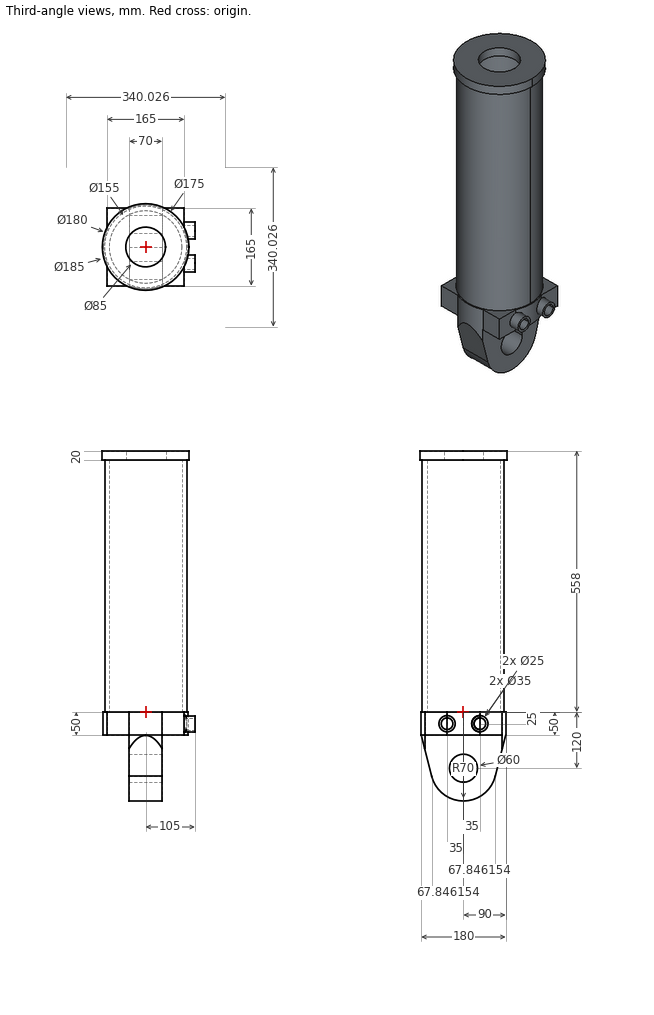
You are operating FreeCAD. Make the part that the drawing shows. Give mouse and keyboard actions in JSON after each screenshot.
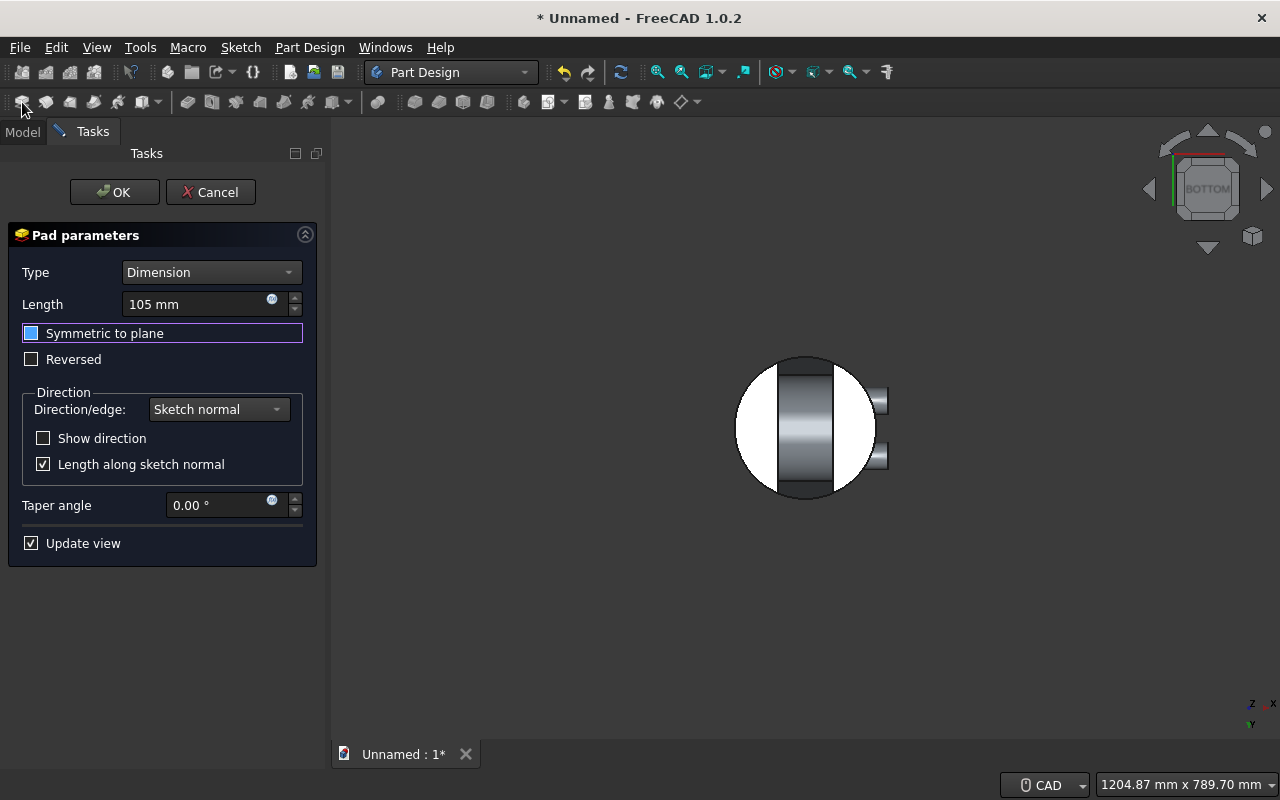
{"action": "left_click", "coordinate": [115, 192]}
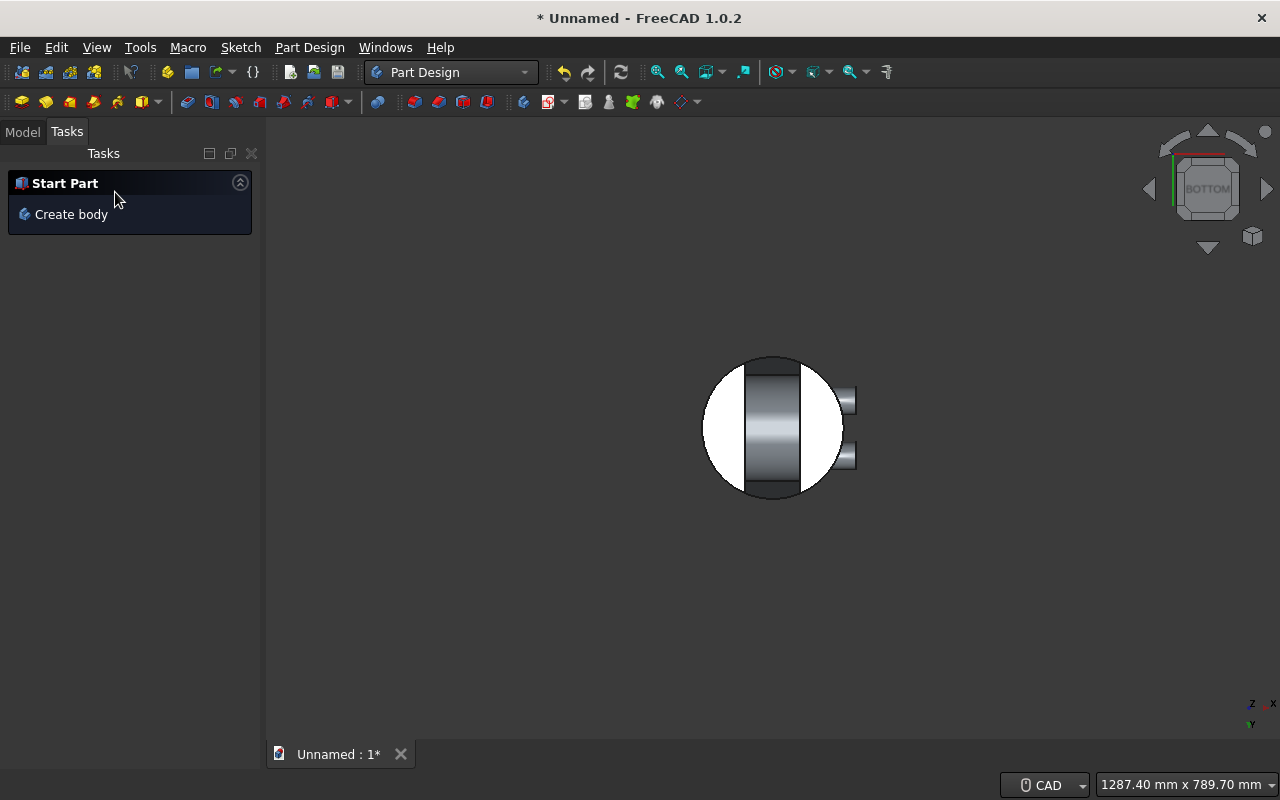
{"action": "left_click", "coordinate": [658, 72]}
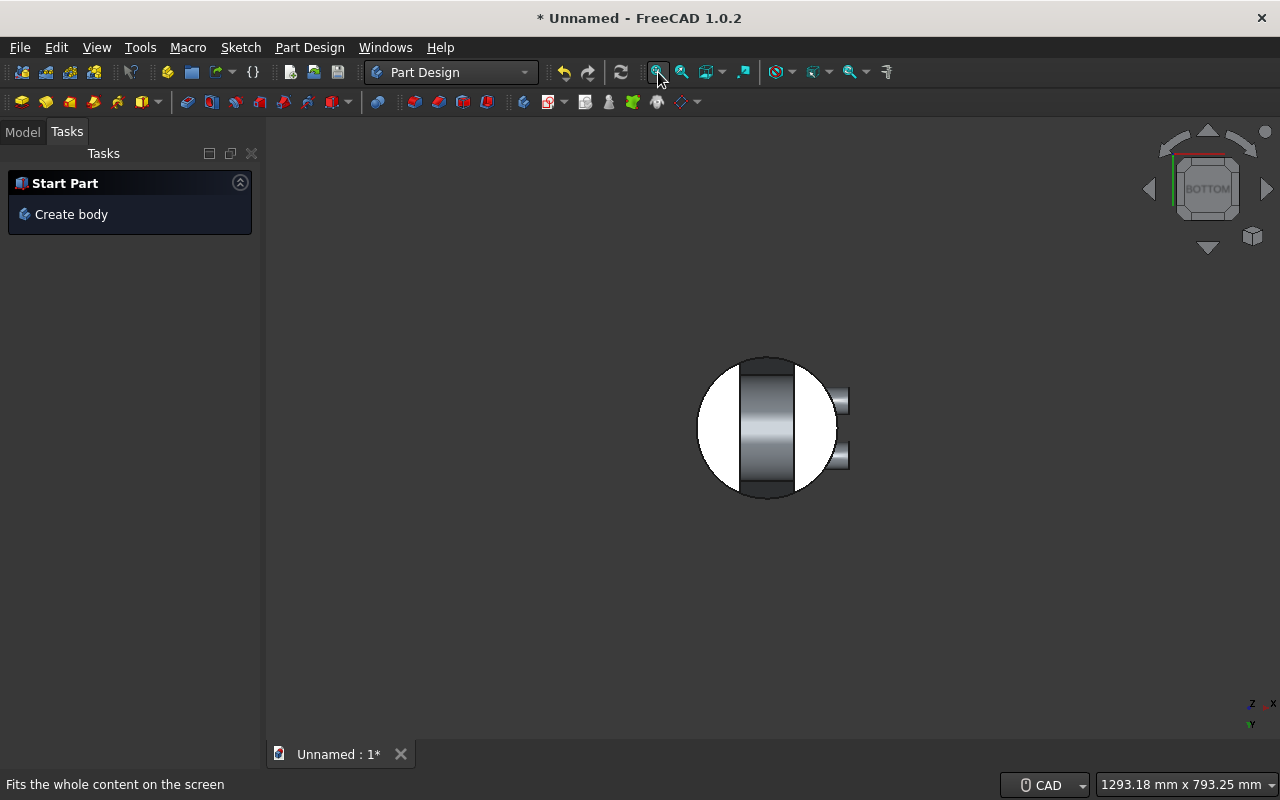
{"action": "key", "text": "0"}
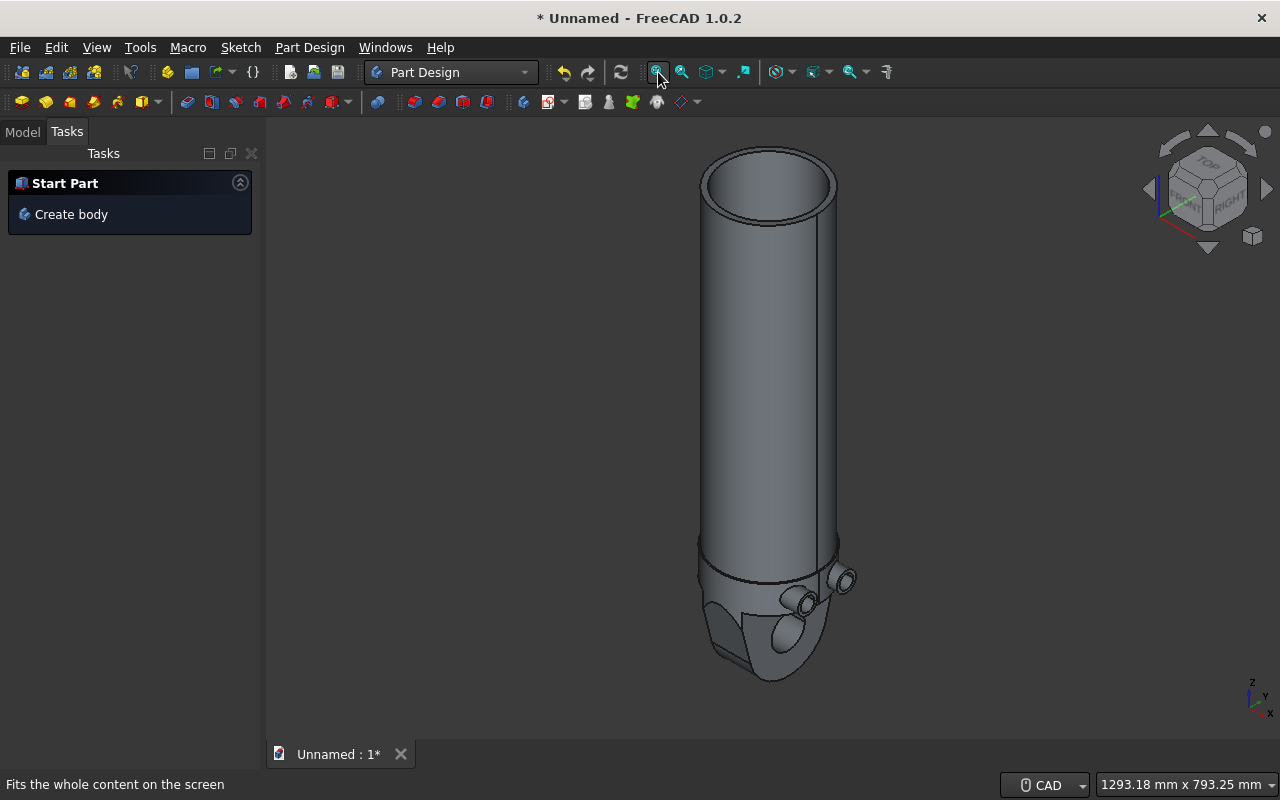
{"action": "scroll", "coordinate": [741, 217], "scroll_direction": "up", "scroll_amount": 12}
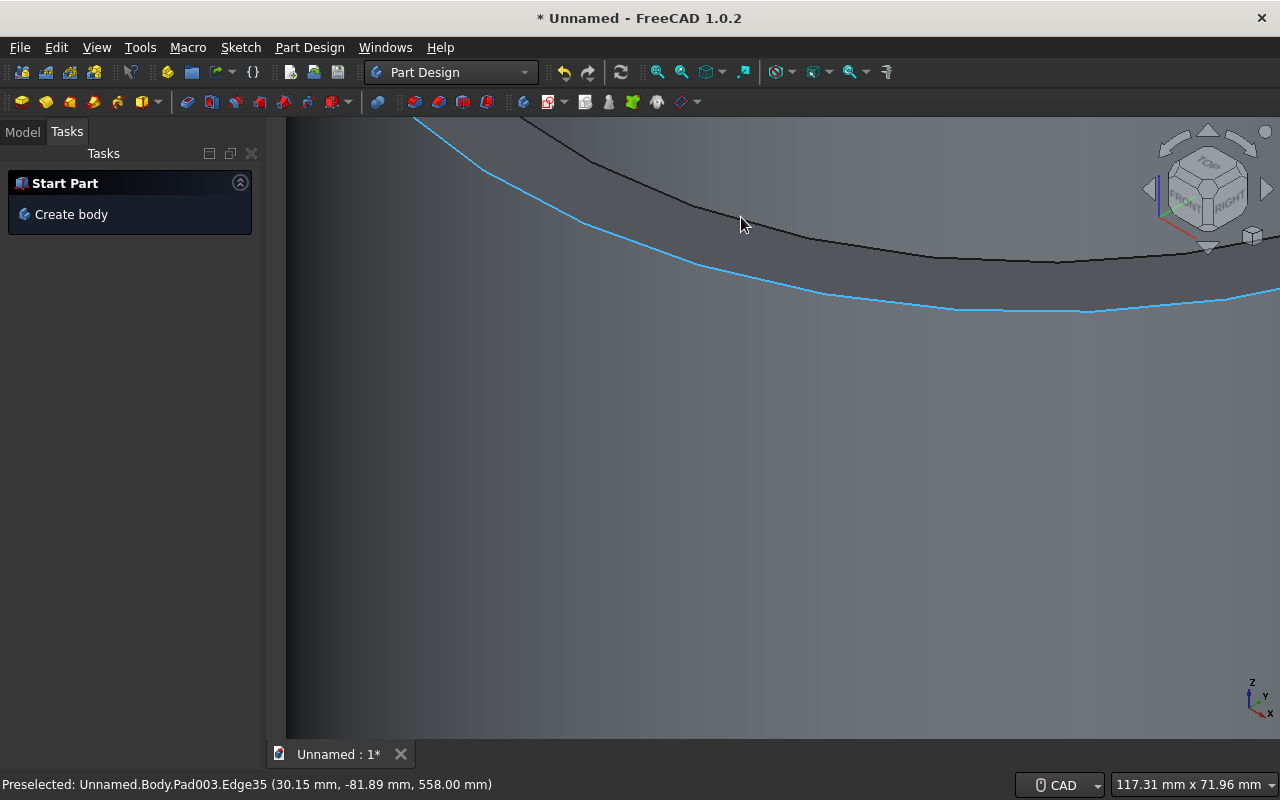
{"action": "left_click", "coordinate": [737, 228]}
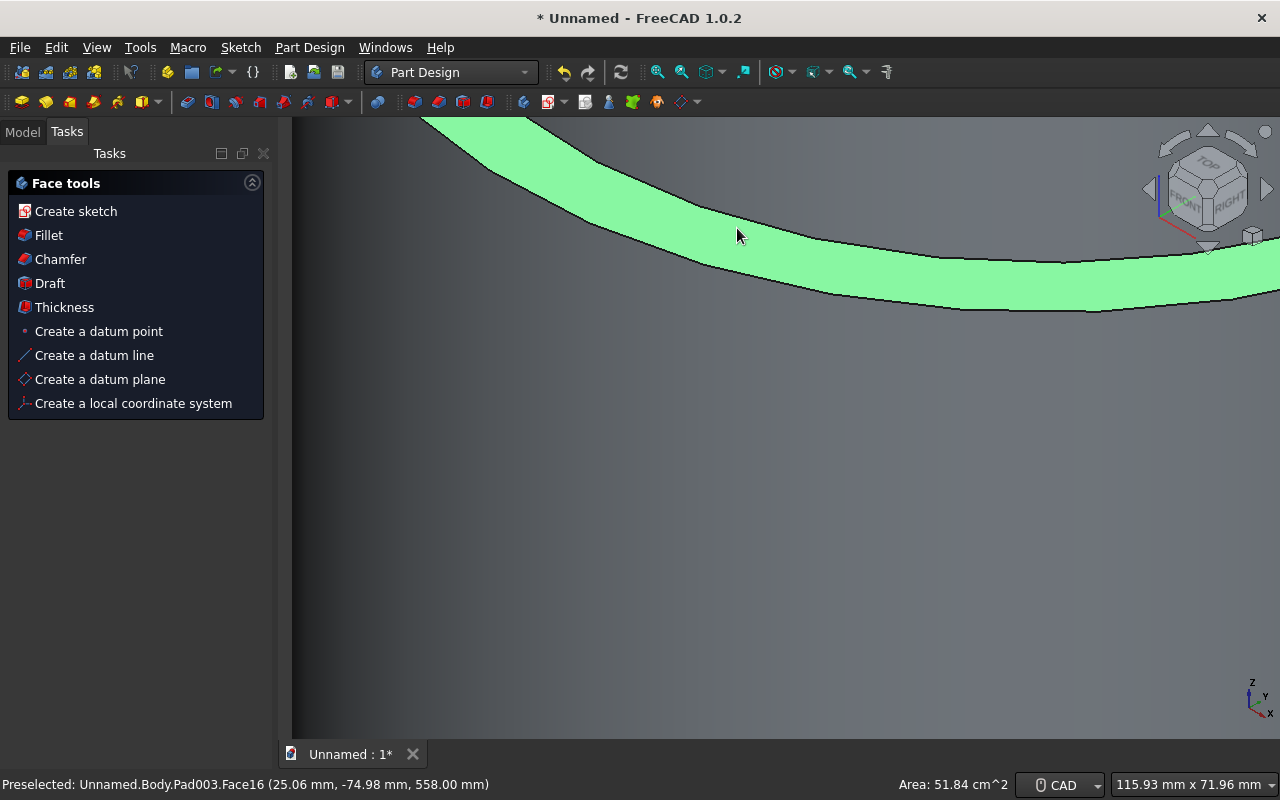
{"action": "left_click", "coordinate": [548, 102]}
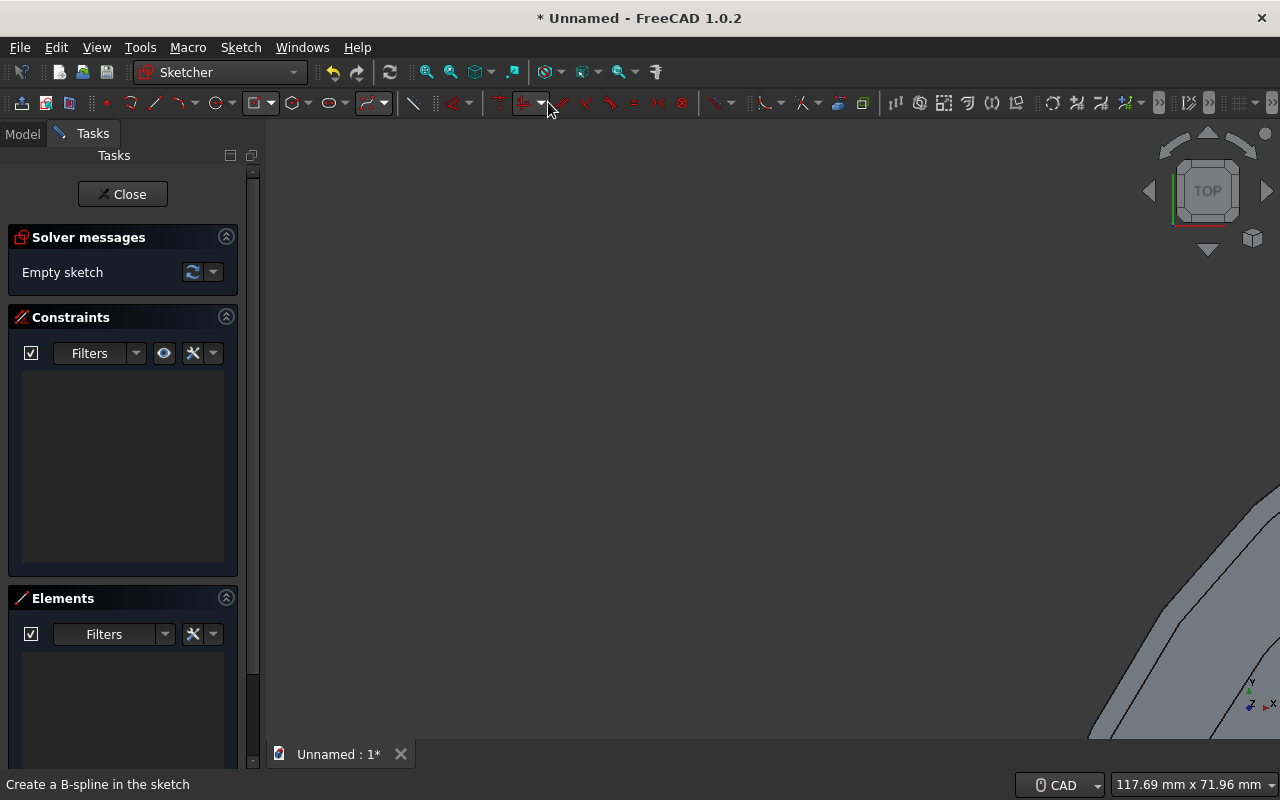
{"action": "scroll", "coordinate": [349, 220], "scroll_direction": "down", "scroll_amount": 7}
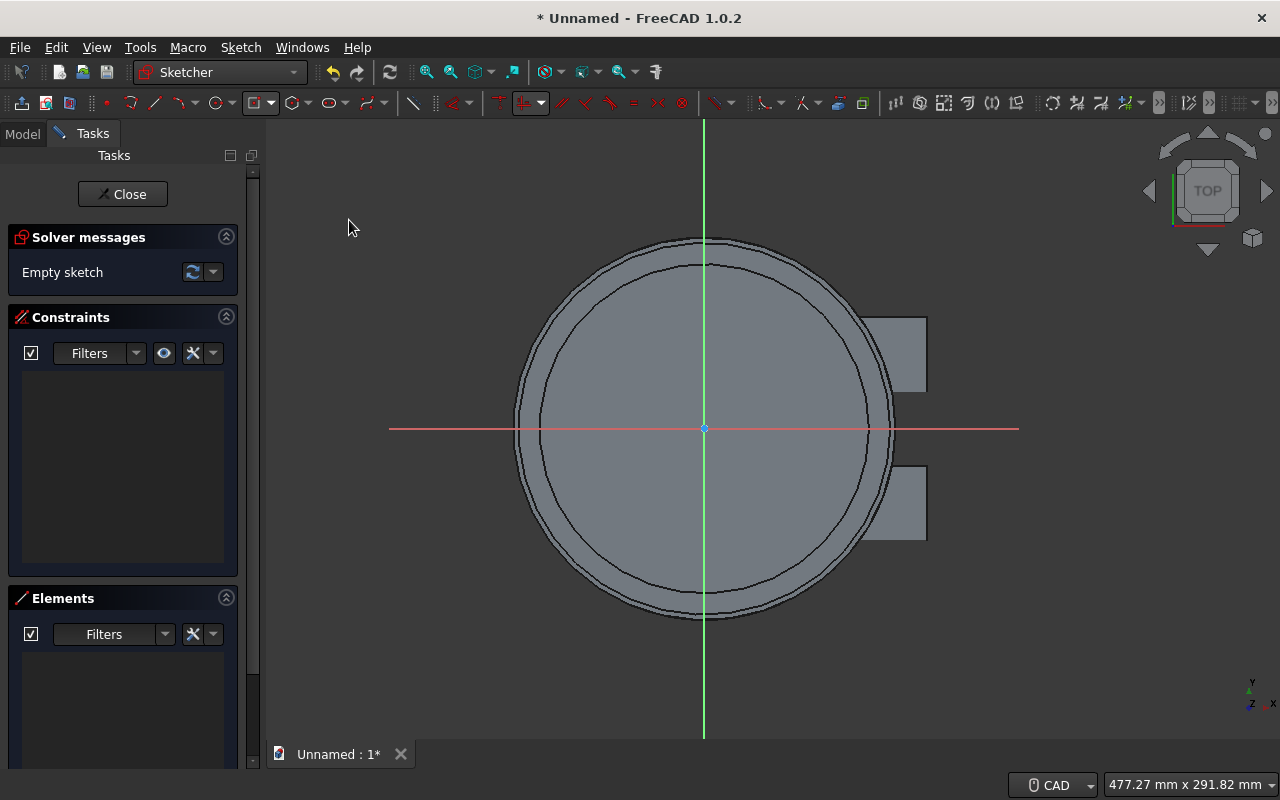
{"action": "left_click", "coordinate": [216, 104]}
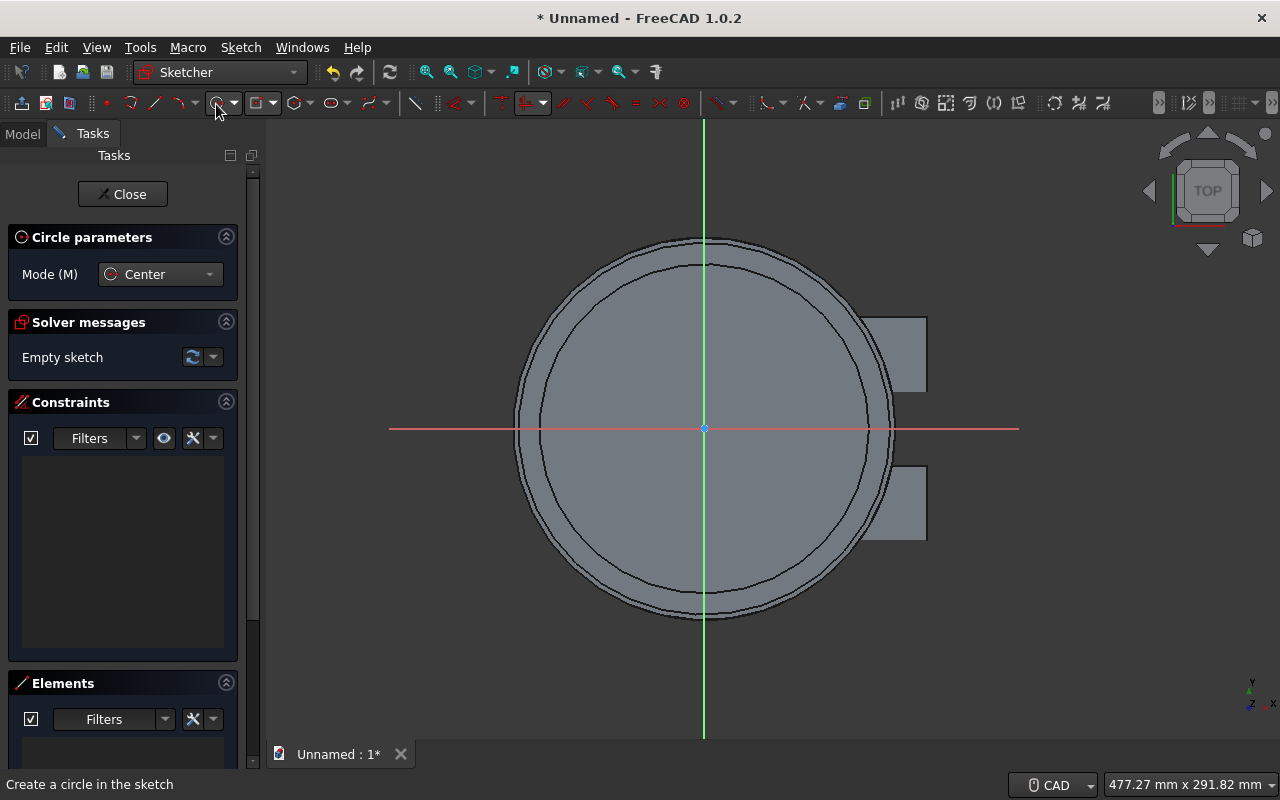
{"action": "left_click", "coordinate": [704, 429]}
{"action": "left_click", "coordinate": [843, 290]}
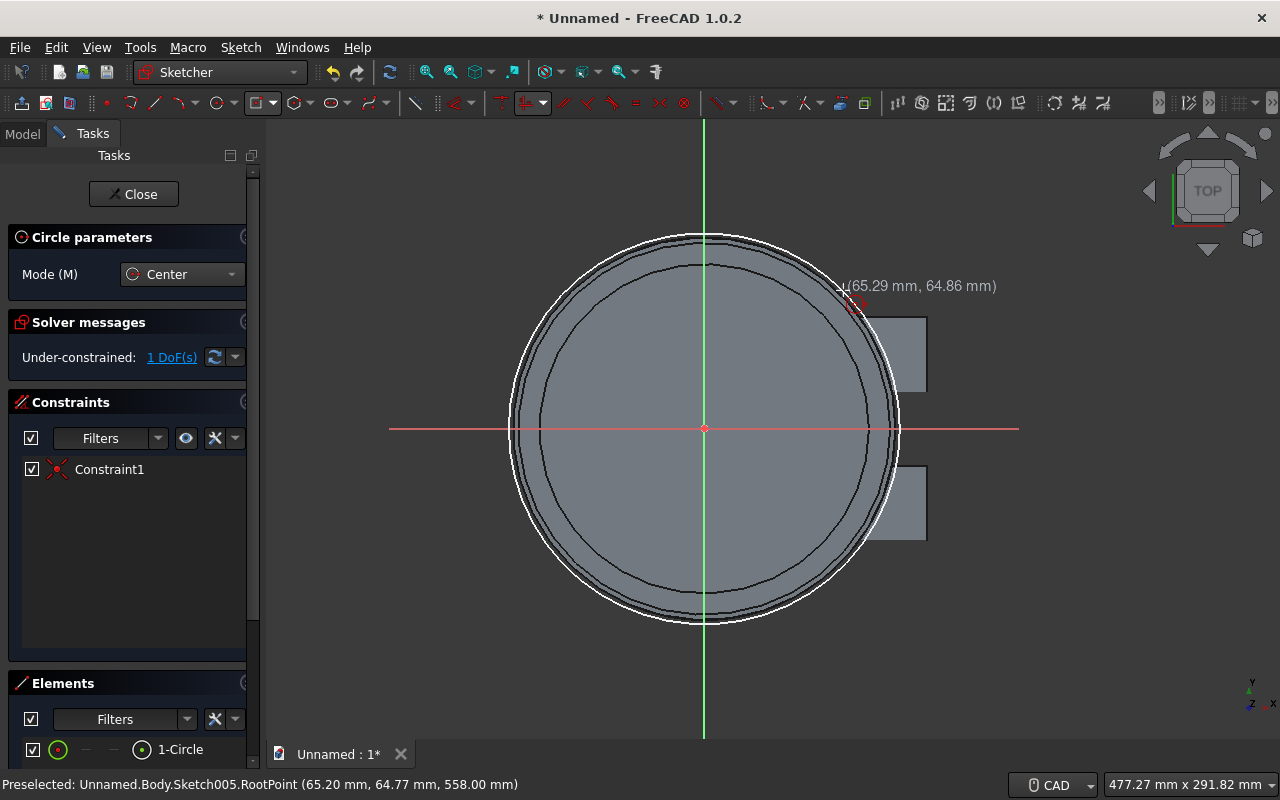
{"action": "left_click", "coordinate": [704, 429]}
{"action": "left_click", "coordinate": [768, 365]}
{"action": "key", "text": "Escape"}